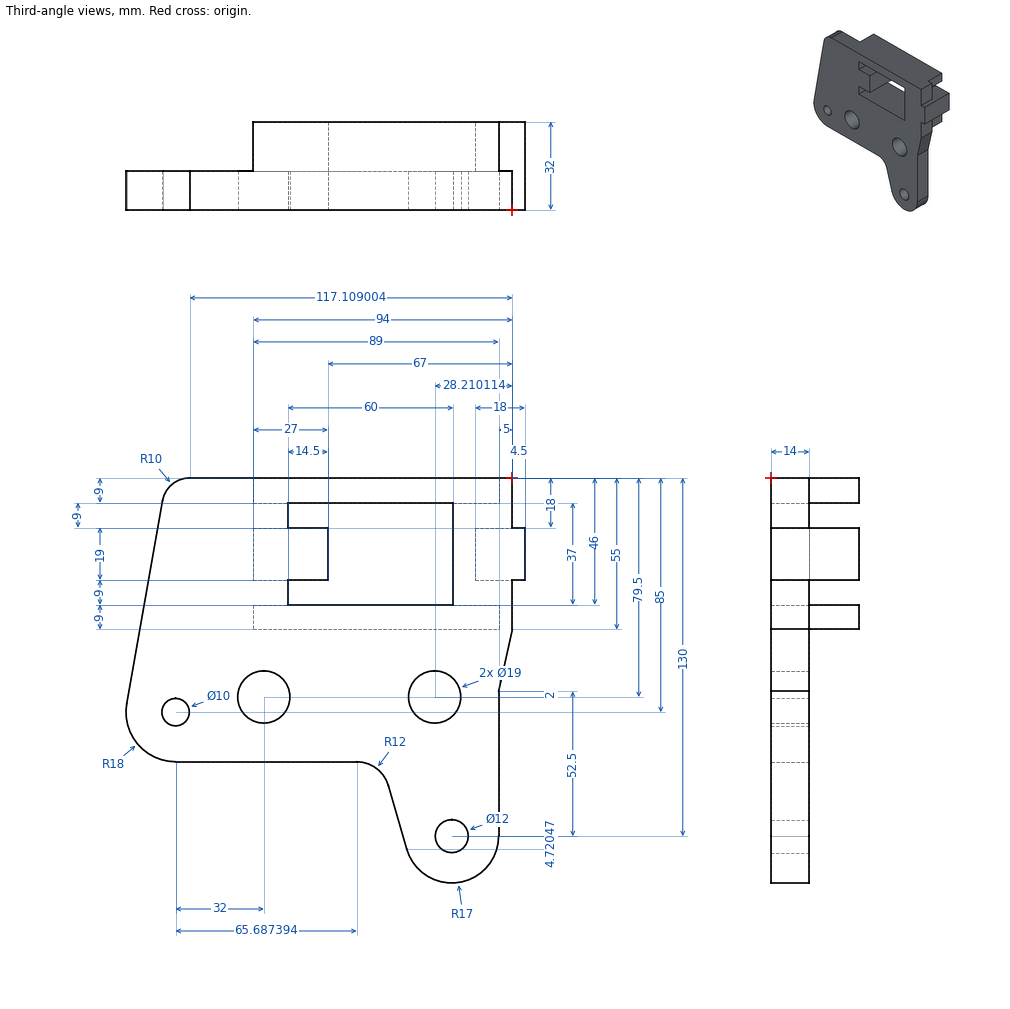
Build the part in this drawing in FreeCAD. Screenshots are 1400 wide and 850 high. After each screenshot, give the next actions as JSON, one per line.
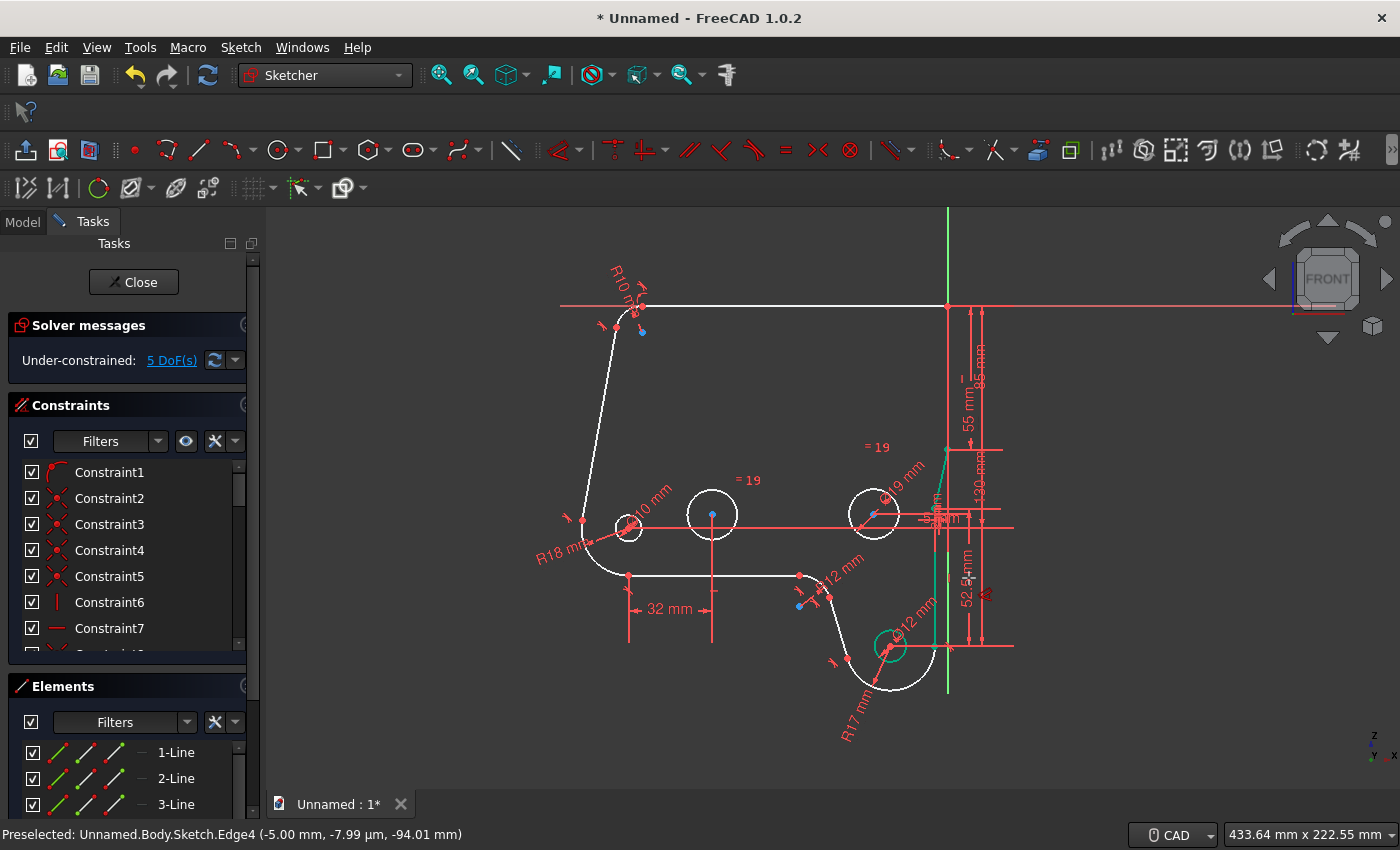
{"action": "left_click", "coordinate": [712, 515]}
{"action": "left_click", "coordinate": [982, 337]}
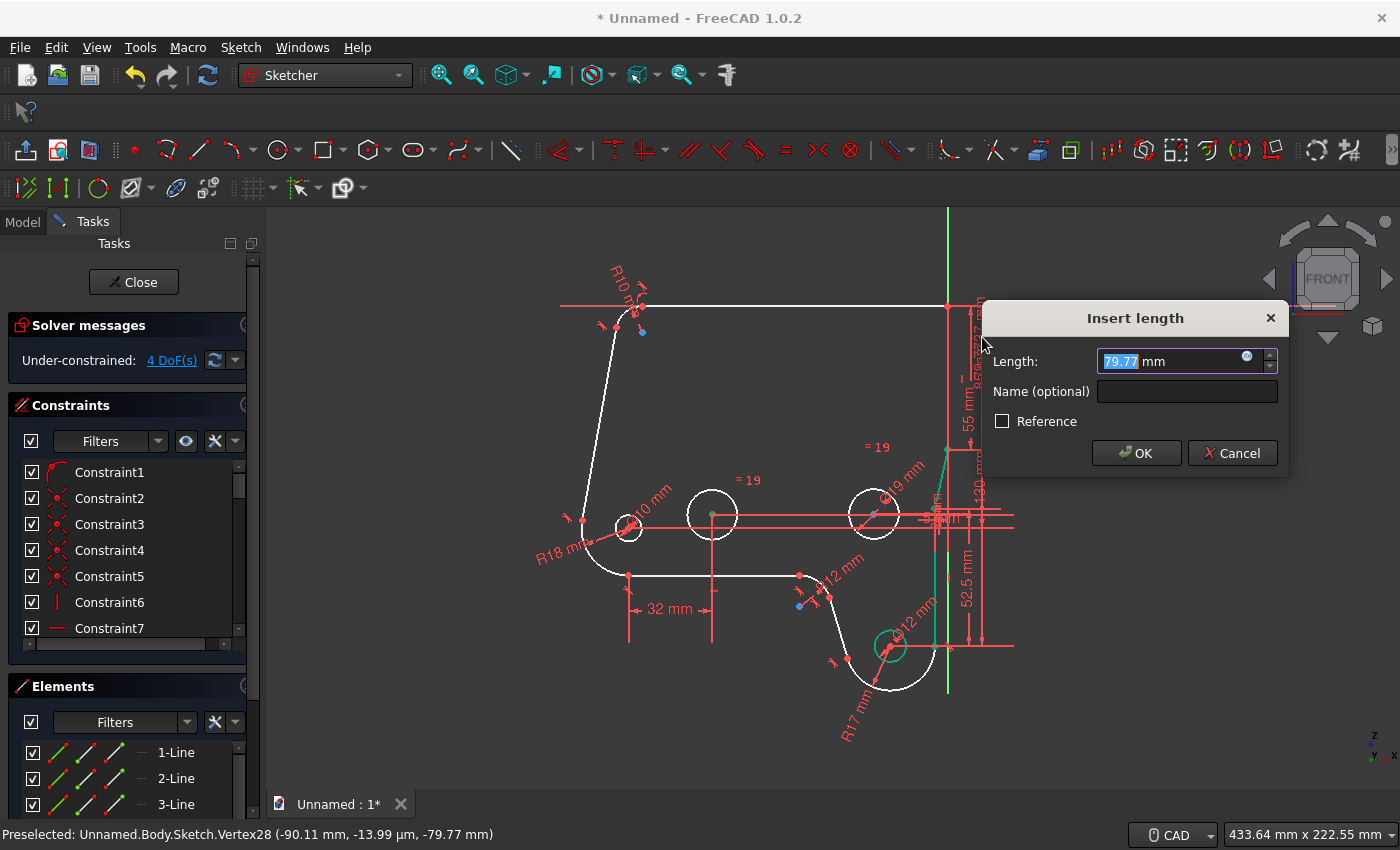
{"action": "type", "text": "79.5"}
{"action": "key", "text": "Return"}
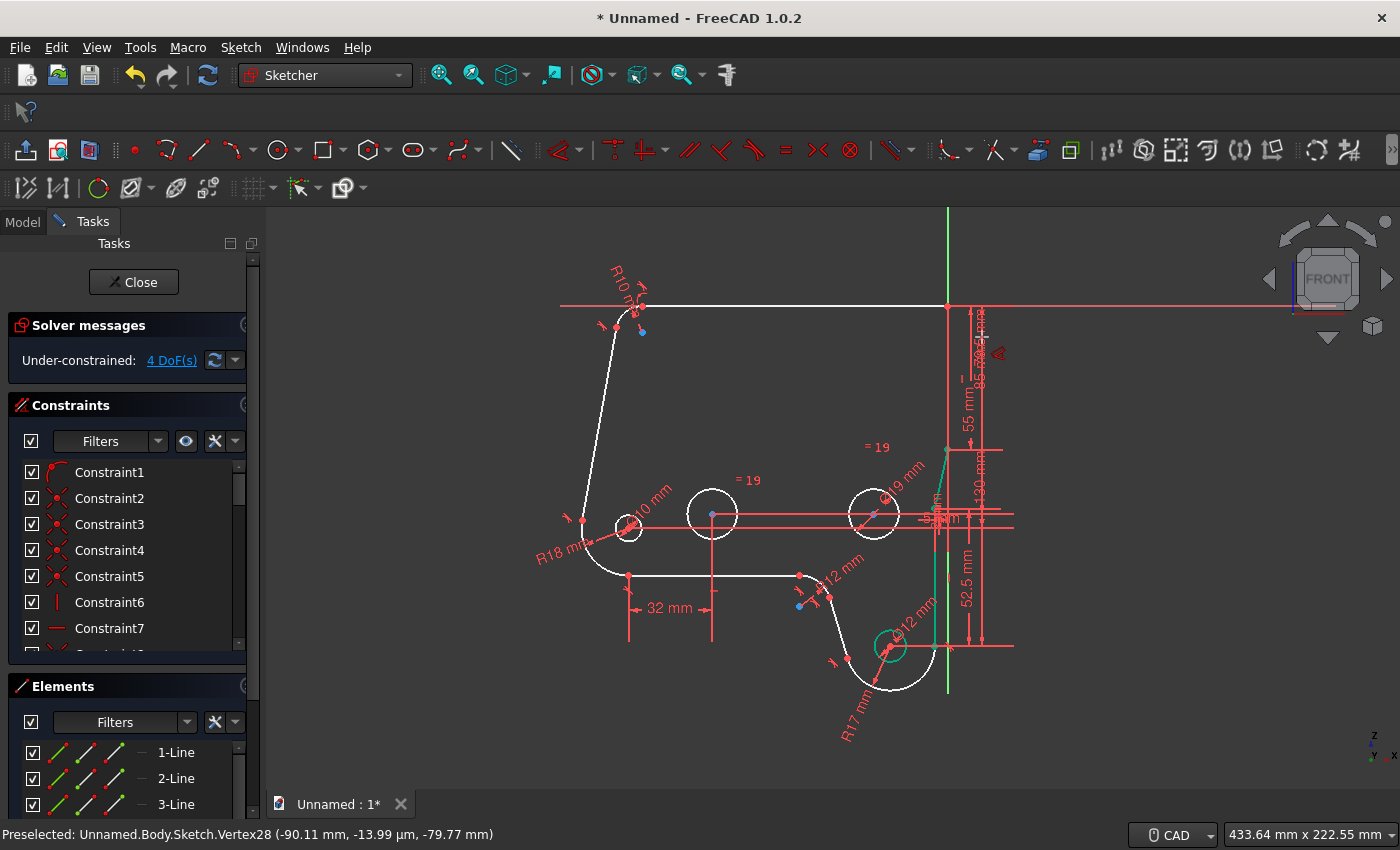
{"action": "scroll", "coordinate": [848, 659], "scroll_direction": "up", "scroll_amount": 6}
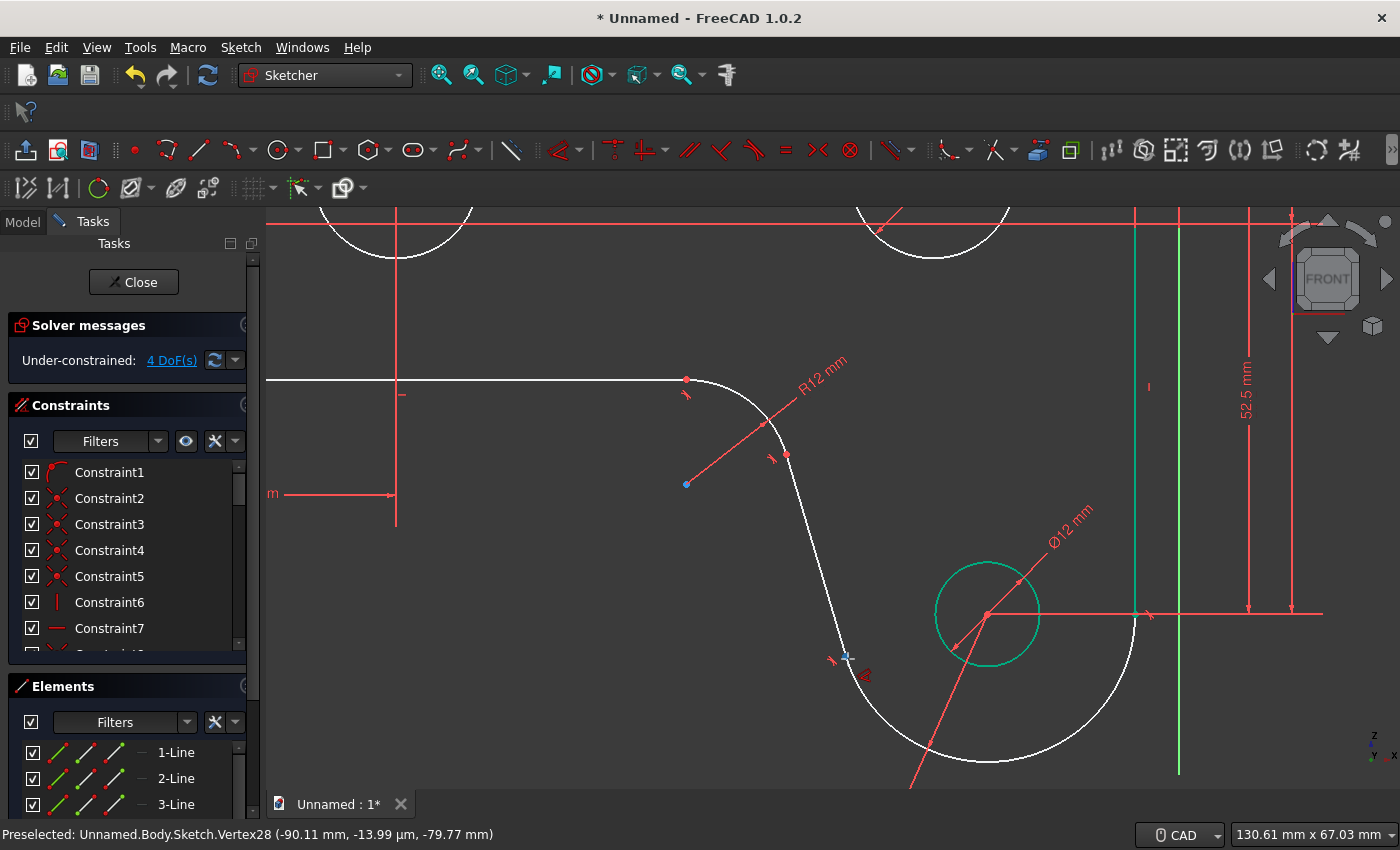
{"action": "left_click", "coordinate": [846, 656]}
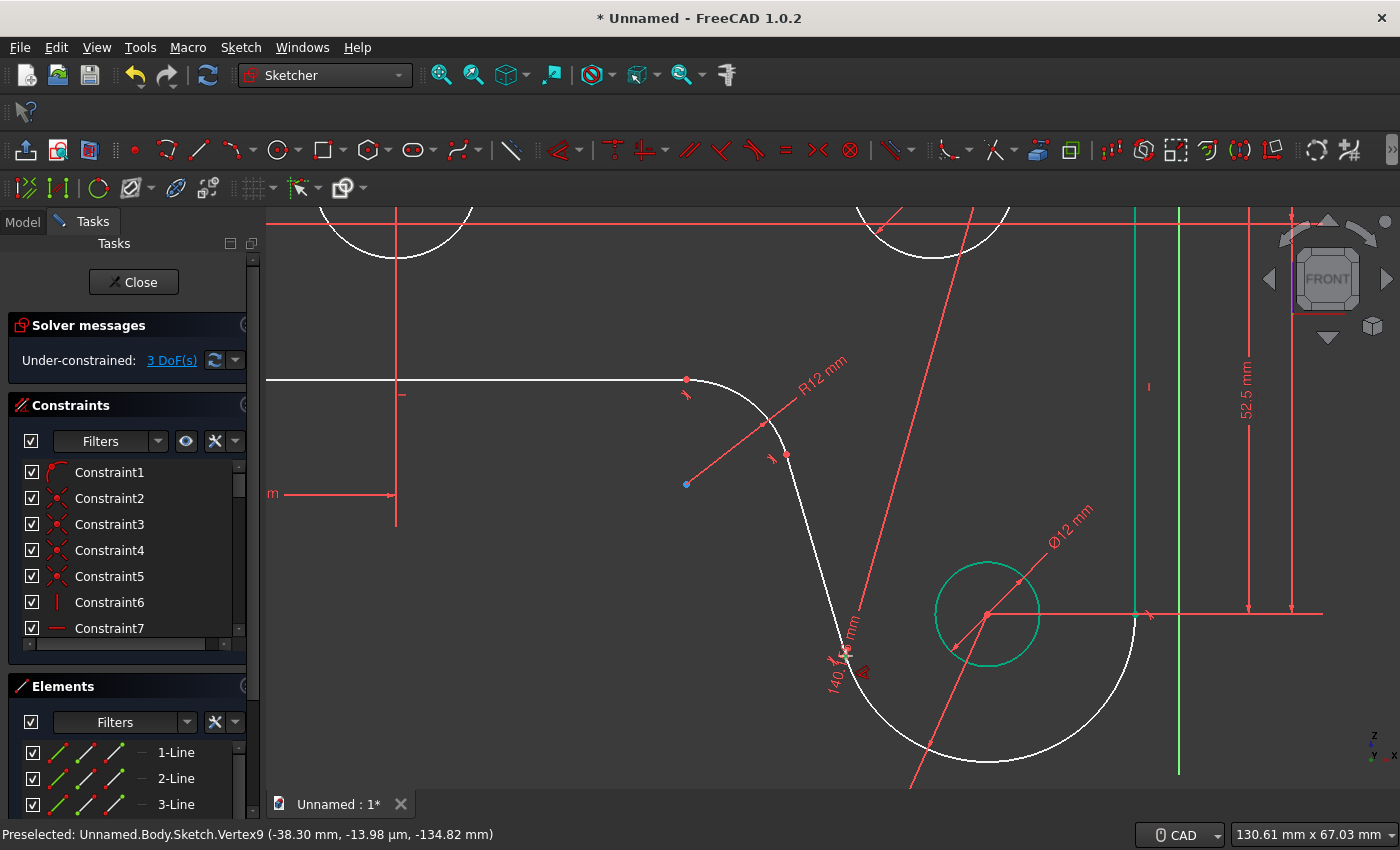
{"action": "left_click", "coordinate": [988, 614]}
{"action": "left_click", "coordinate": [1022, 626]}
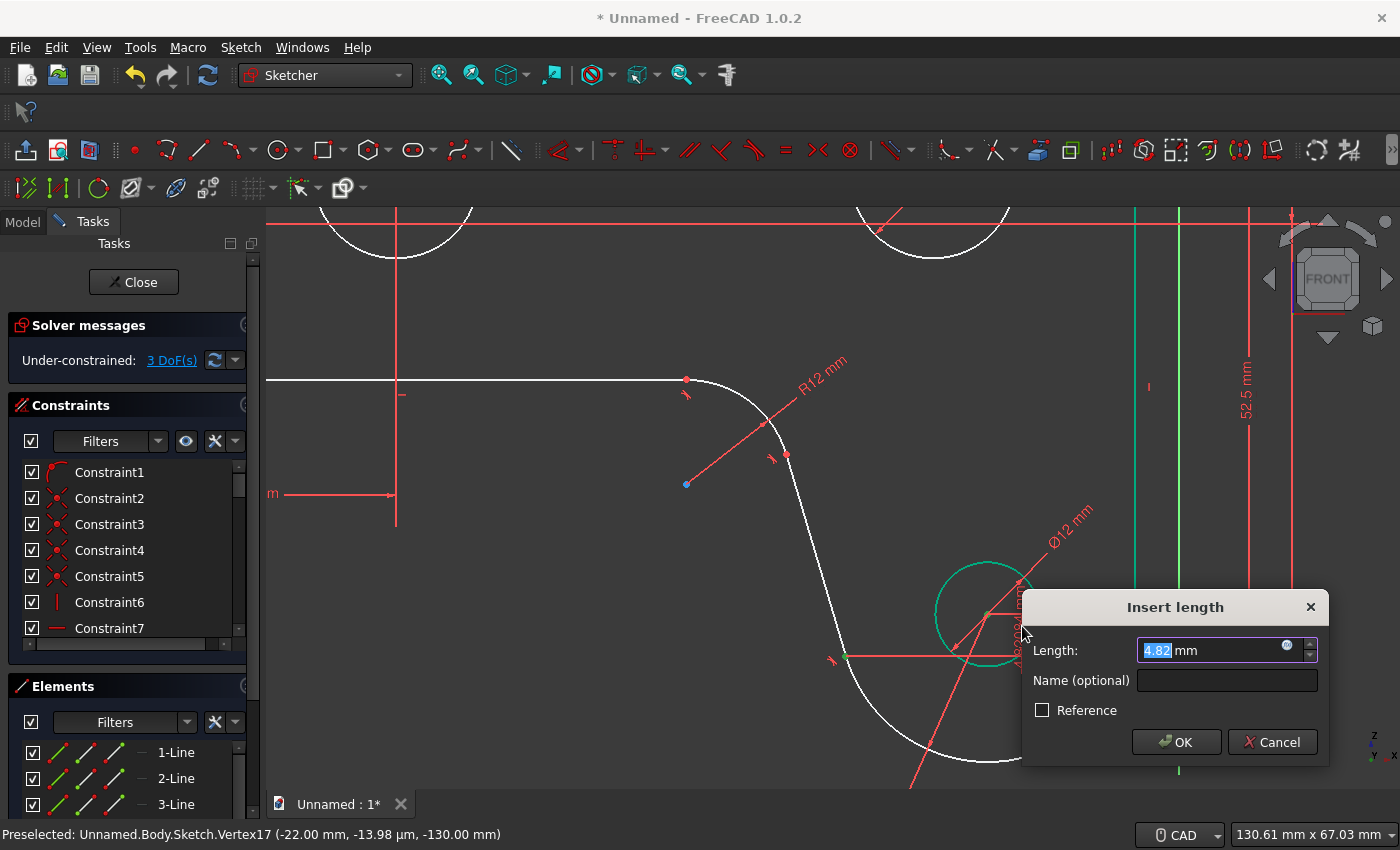
{"action": "type", "text": "4.72047"}
{"action": "key", "text": "Return"}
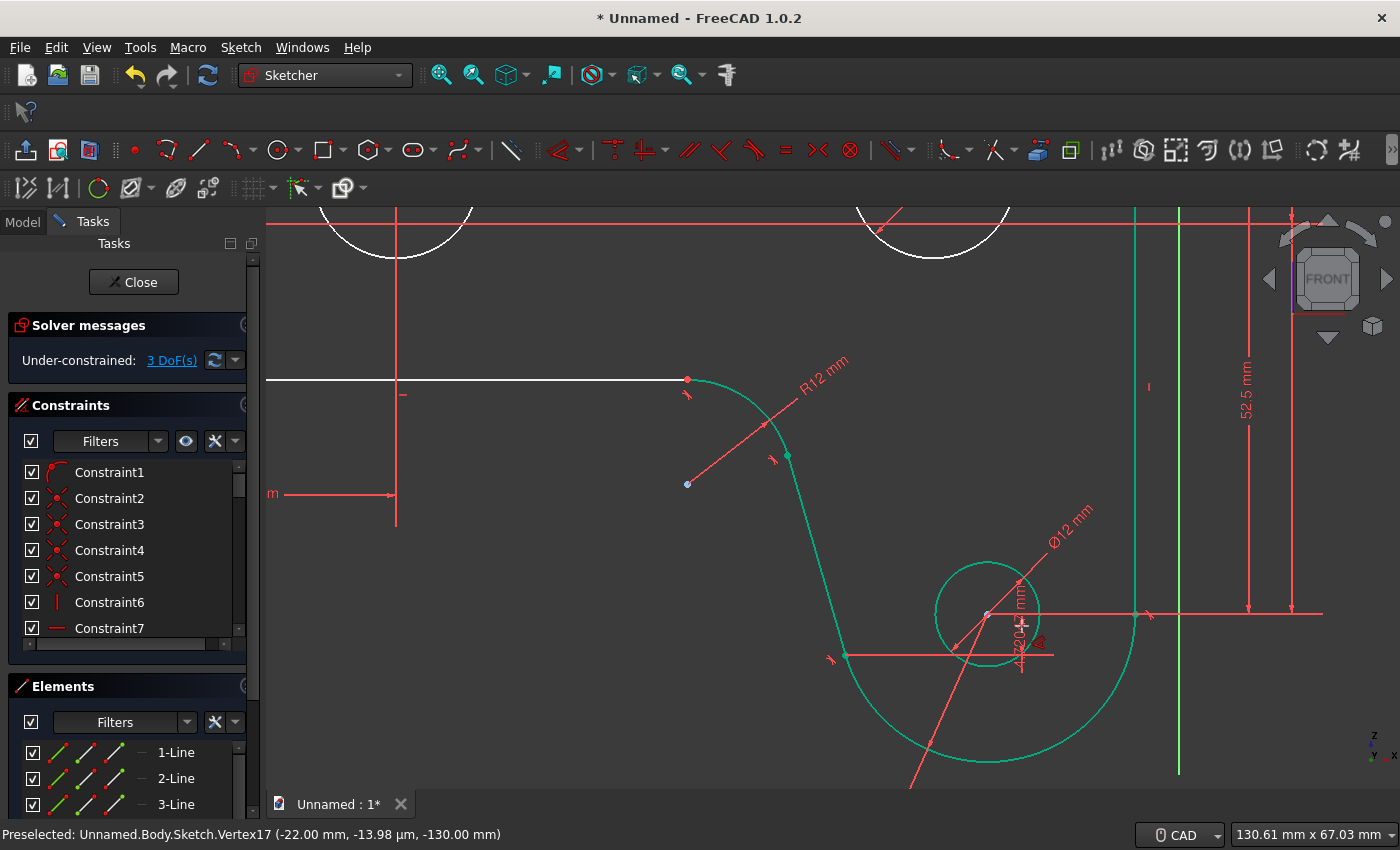
{"action": "scroll", "coordinate": [848, 660], "scroll_direction": "down", "scroll_amount": 6}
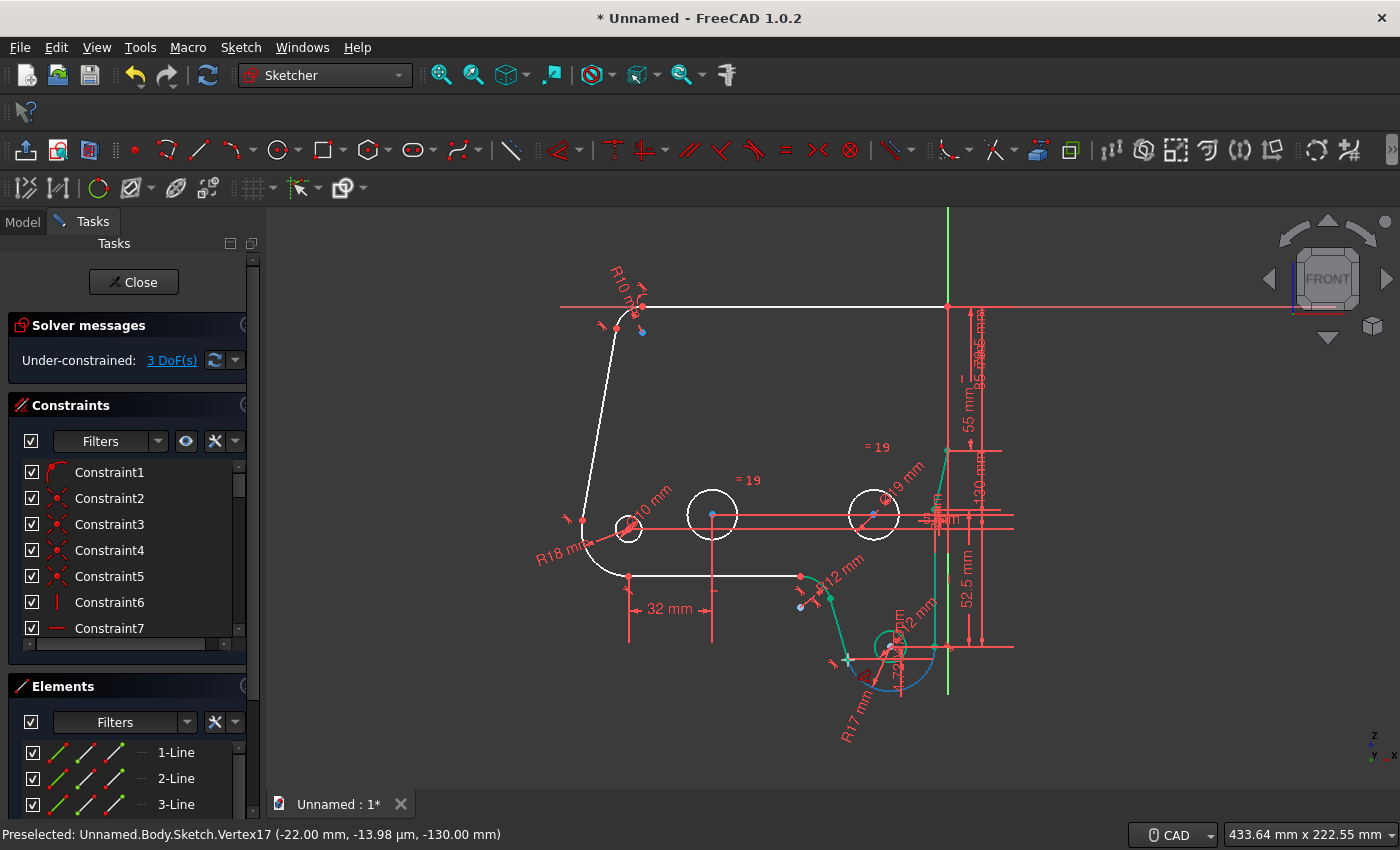
{"action": "left_click", "coordinate": [749, 576]}
{"action": "left_click", "coordinate": [754, 610]}